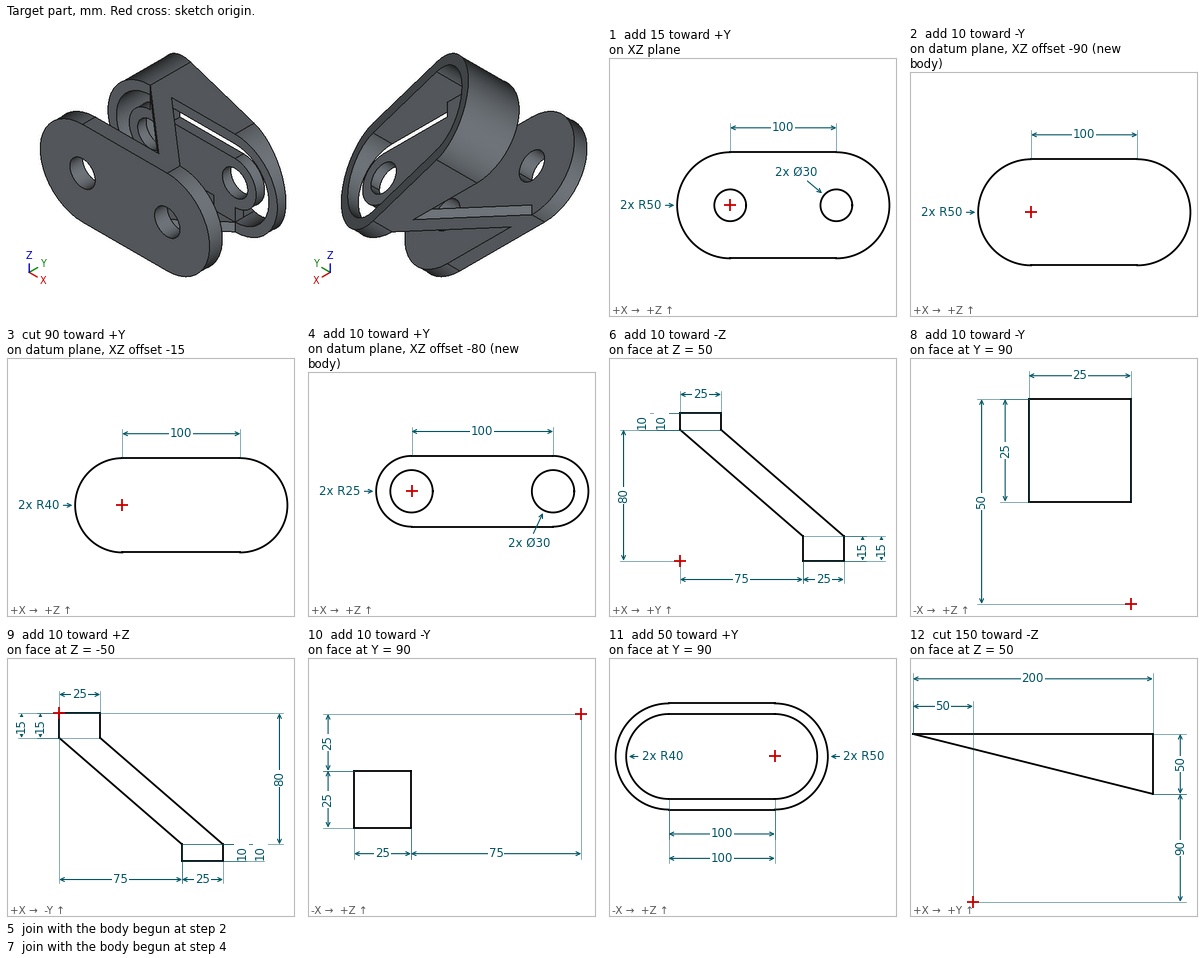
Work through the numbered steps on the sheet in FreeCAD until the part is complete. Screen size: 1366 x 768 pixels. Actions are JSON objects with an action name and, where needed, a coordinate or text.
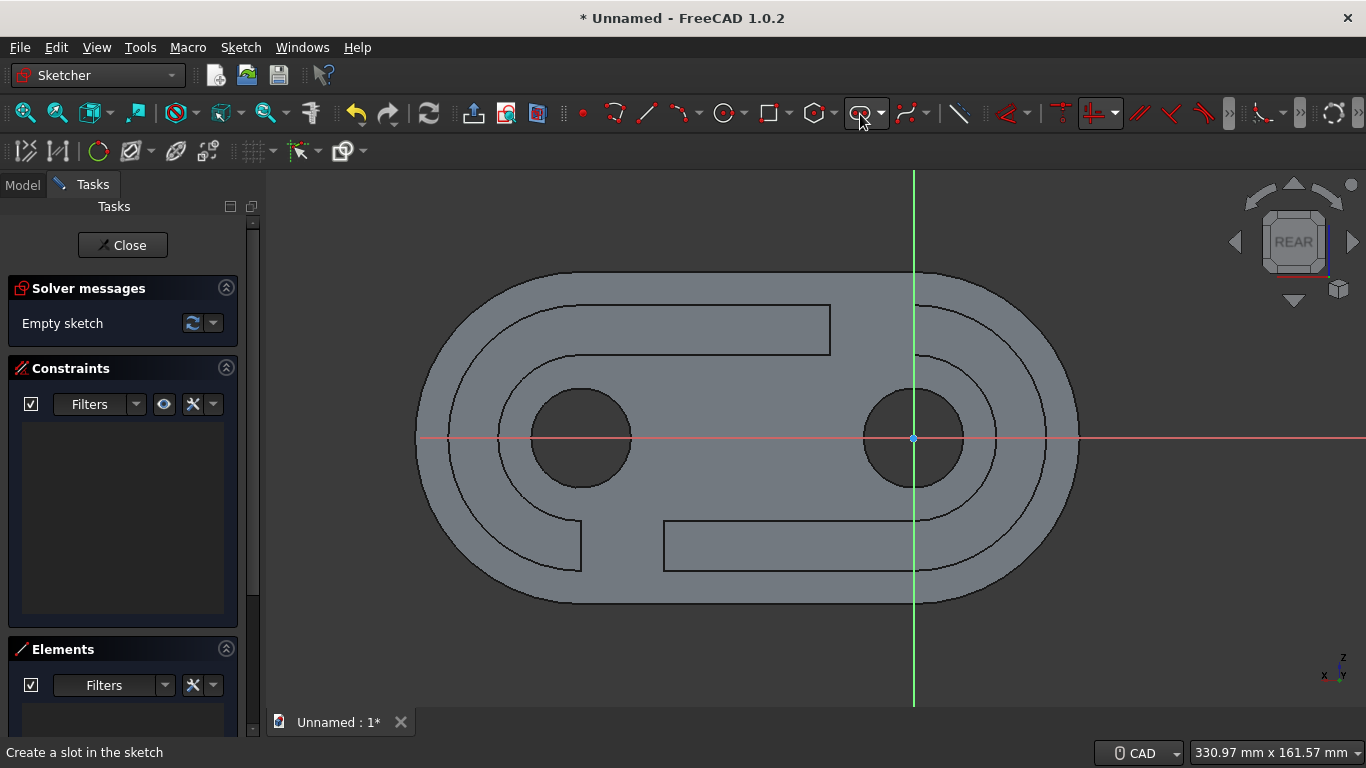
{"action": "left_click", "coordinate": [914, 438]}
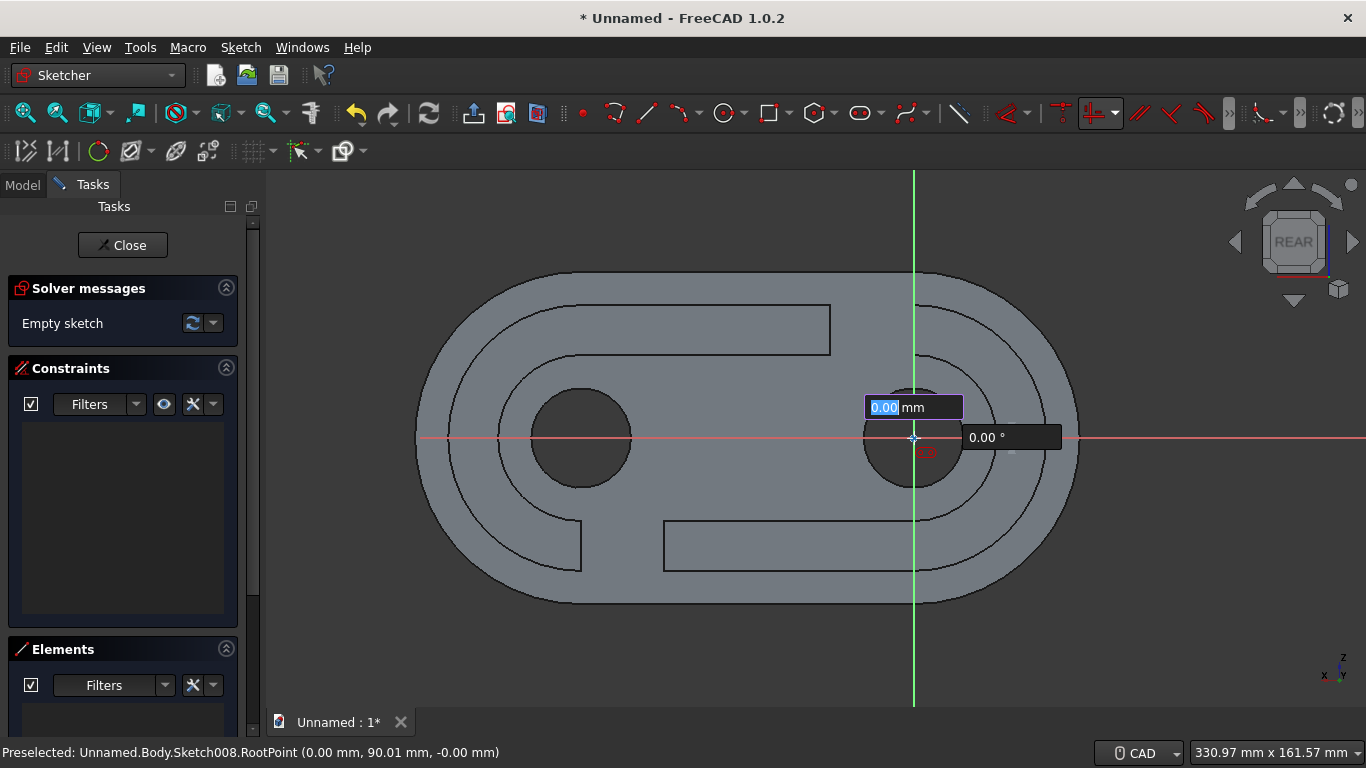
{"action": "left_click", "coordinate": [581, 429]}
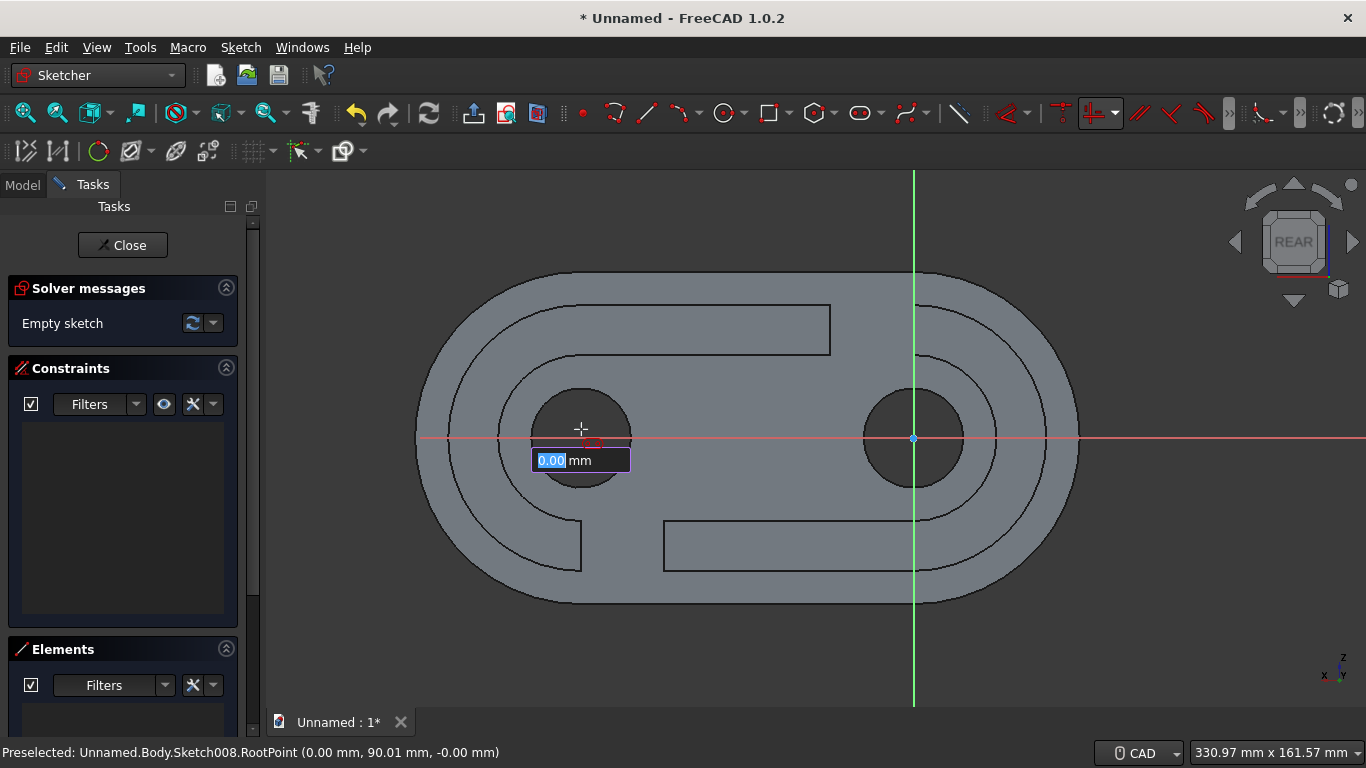
{"action": "left_click", "coordinate": [747, 604]}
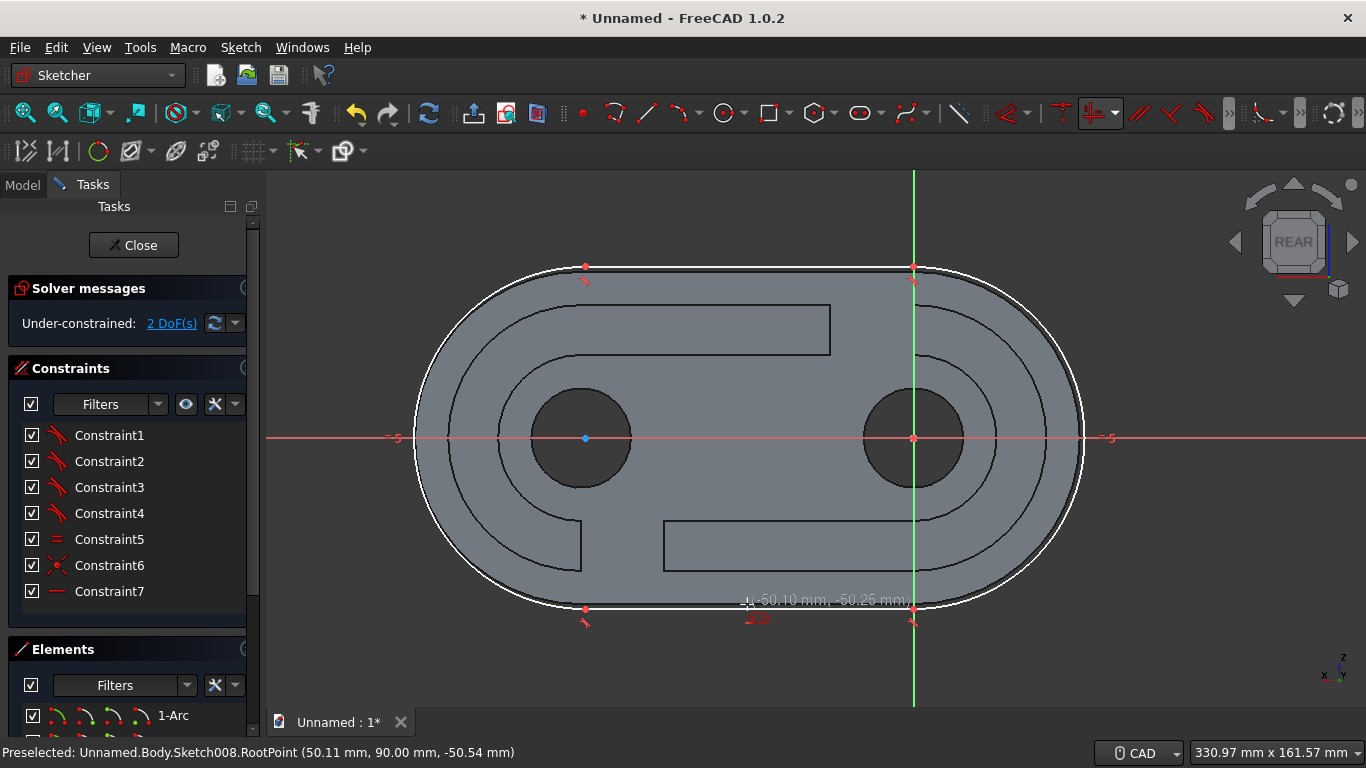
{"action": "left_click", "coordinate": [914, 438]}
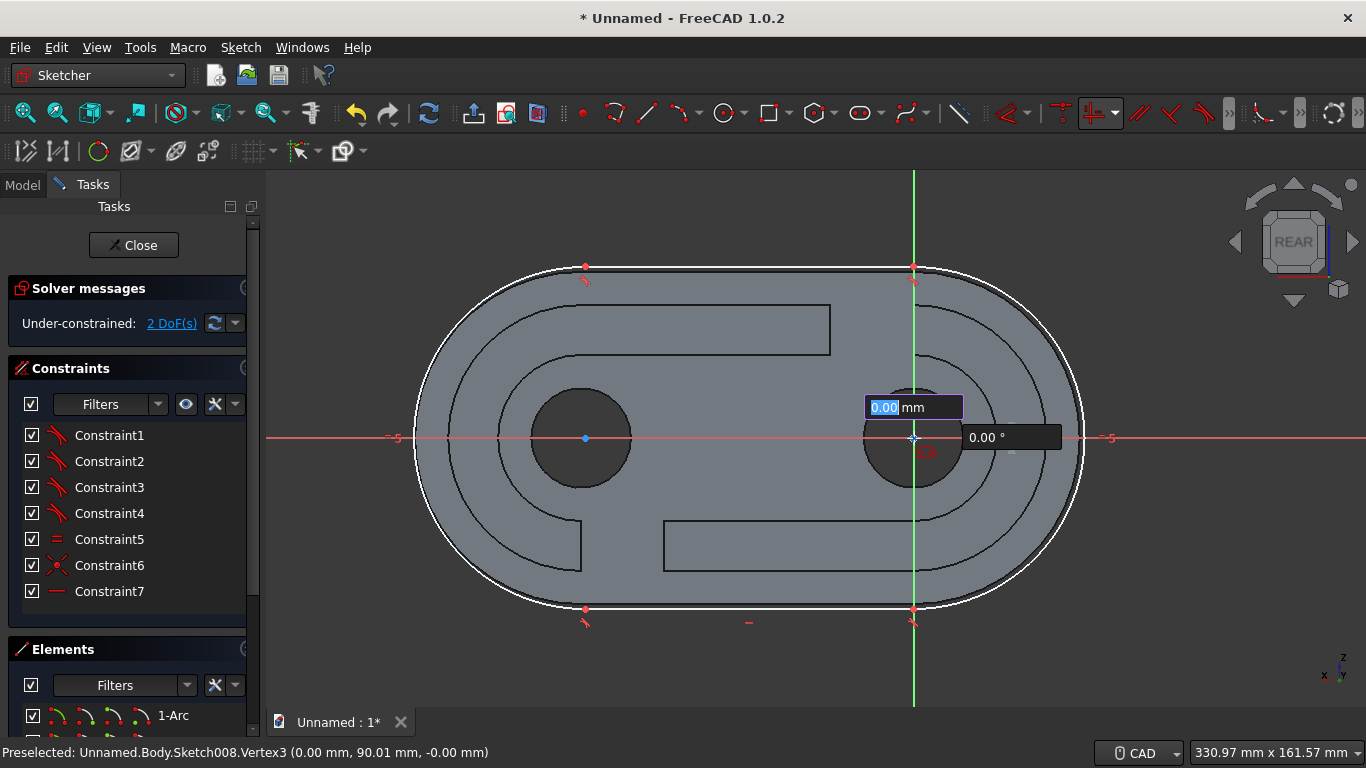
{"action": "left_click", "coordinate": [581, 429]}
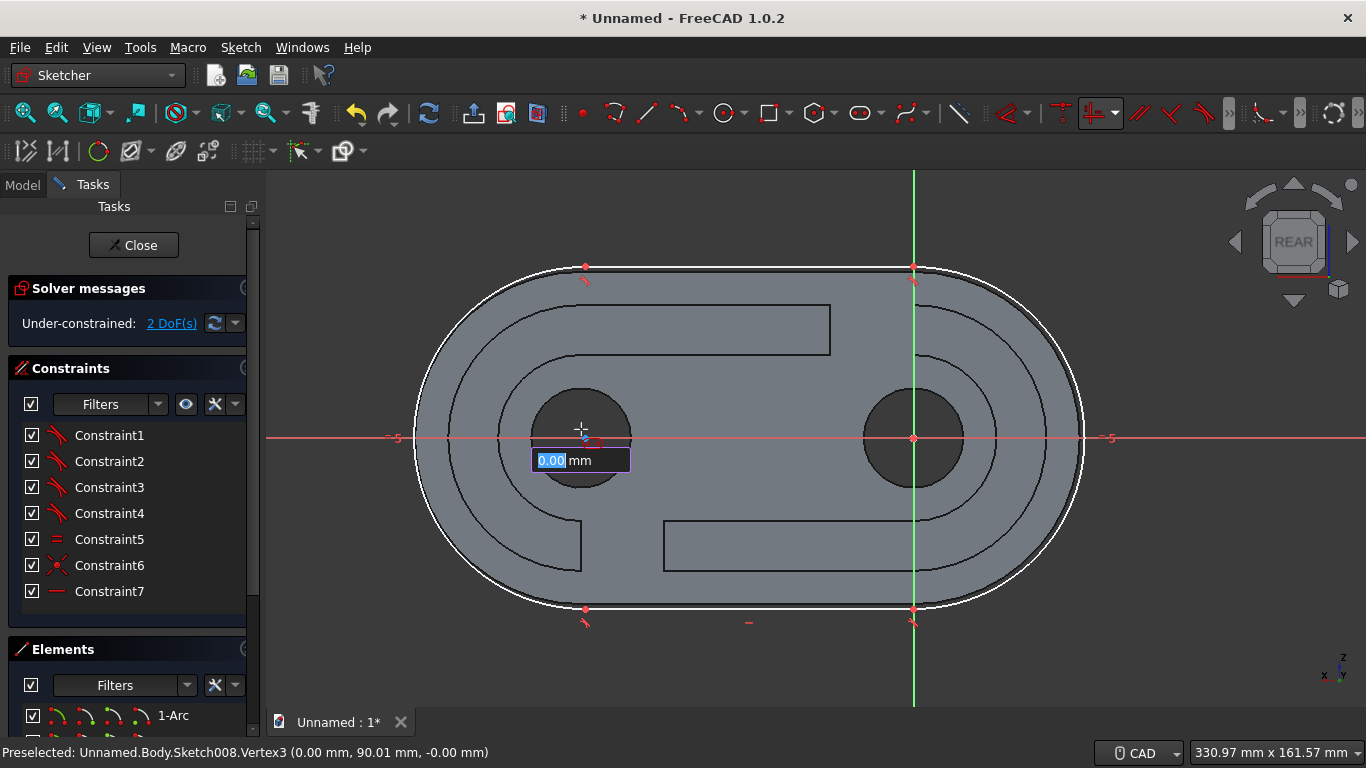
{"action": "left_click", "coordinate": [747, 571]}
{"action": "key", "text": "Escape"}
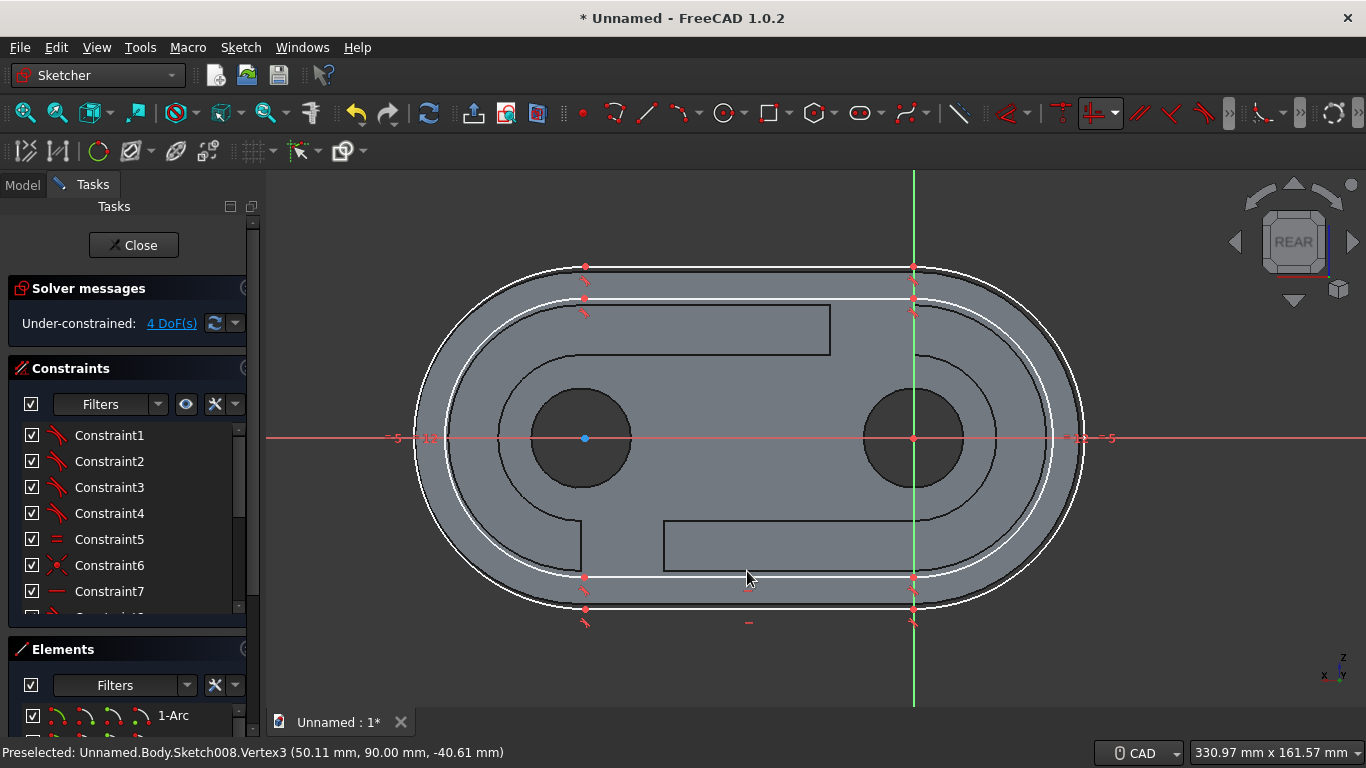
{"action": "left_click", "coordinate": [1006, 114]}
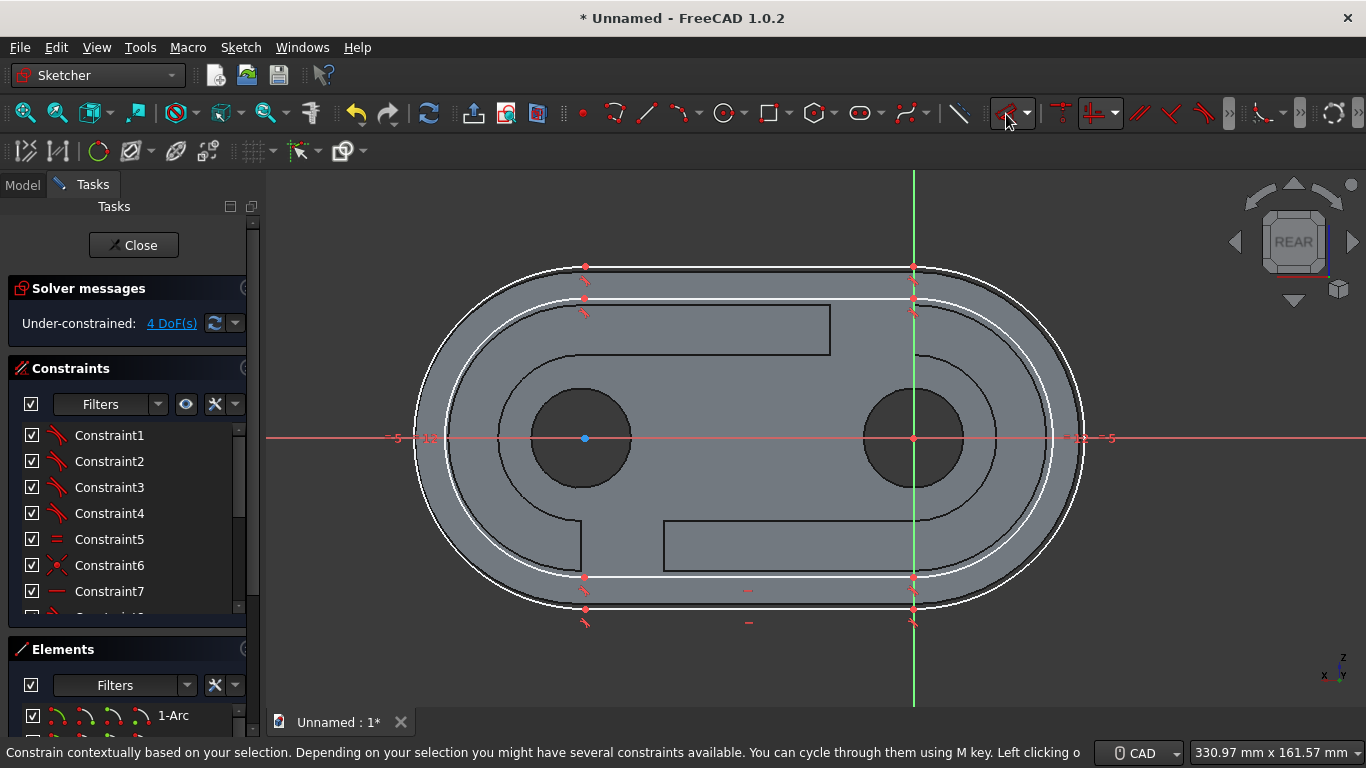
{"action": "left_click", "coordinate": [1052, 539]}
{"action": "left_click", "coordinate": [1078, 558]}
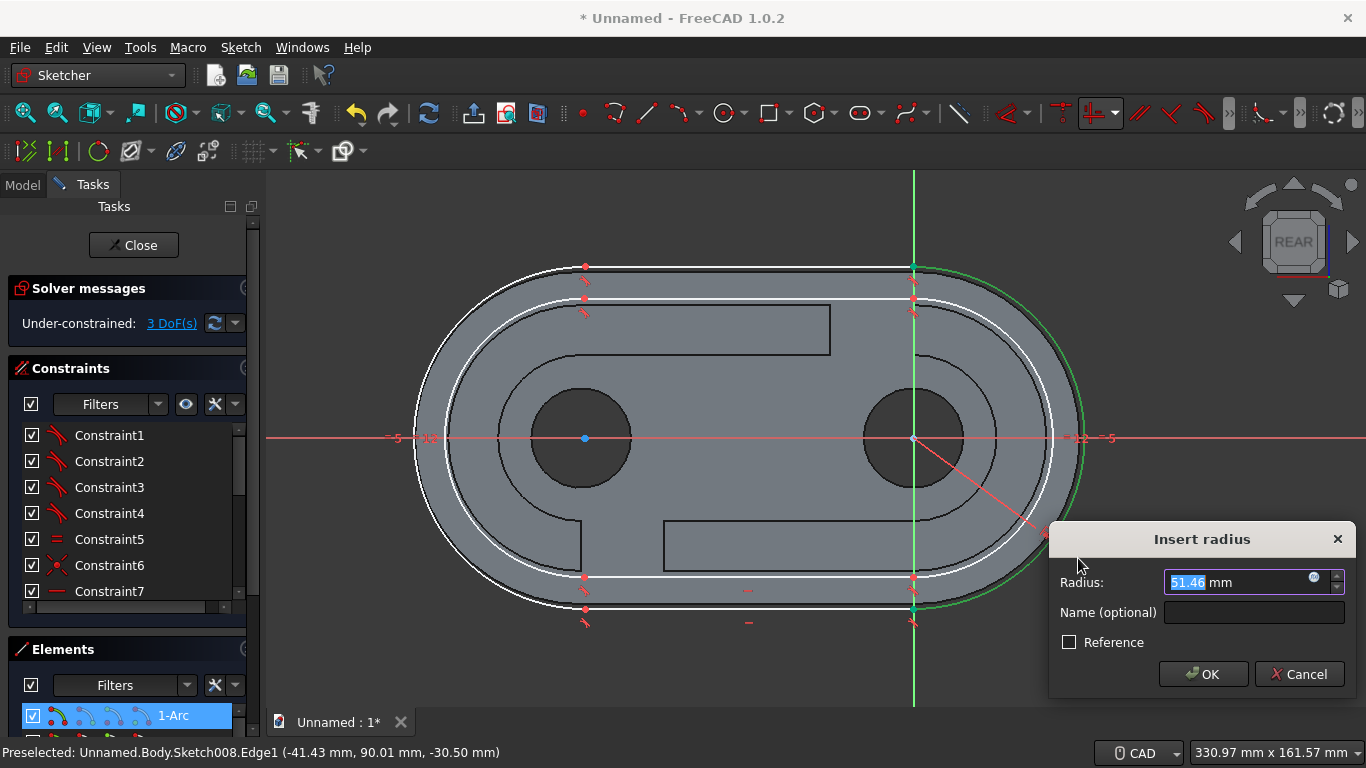
{"action": "type", "text": "50"}
{"action": "key", "text": "Return"}